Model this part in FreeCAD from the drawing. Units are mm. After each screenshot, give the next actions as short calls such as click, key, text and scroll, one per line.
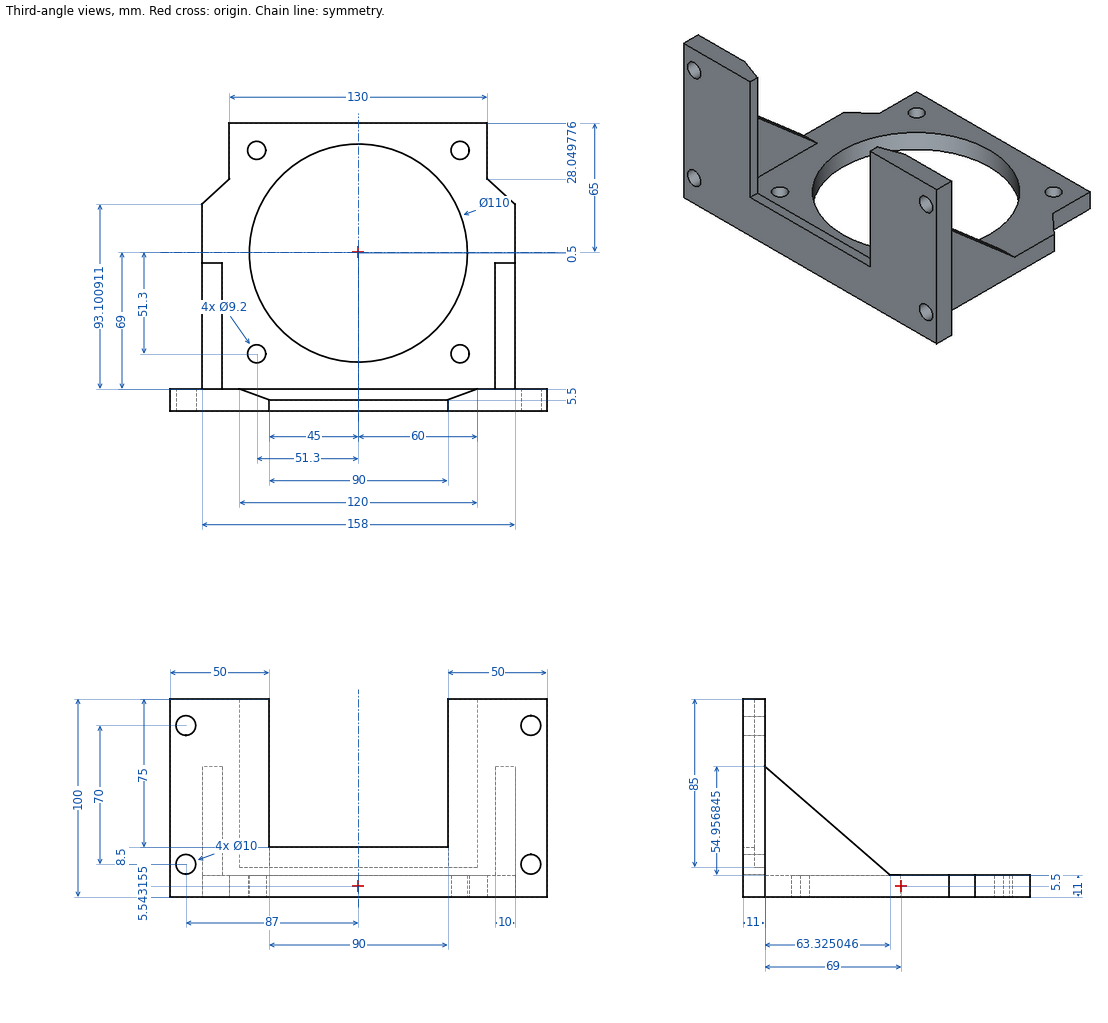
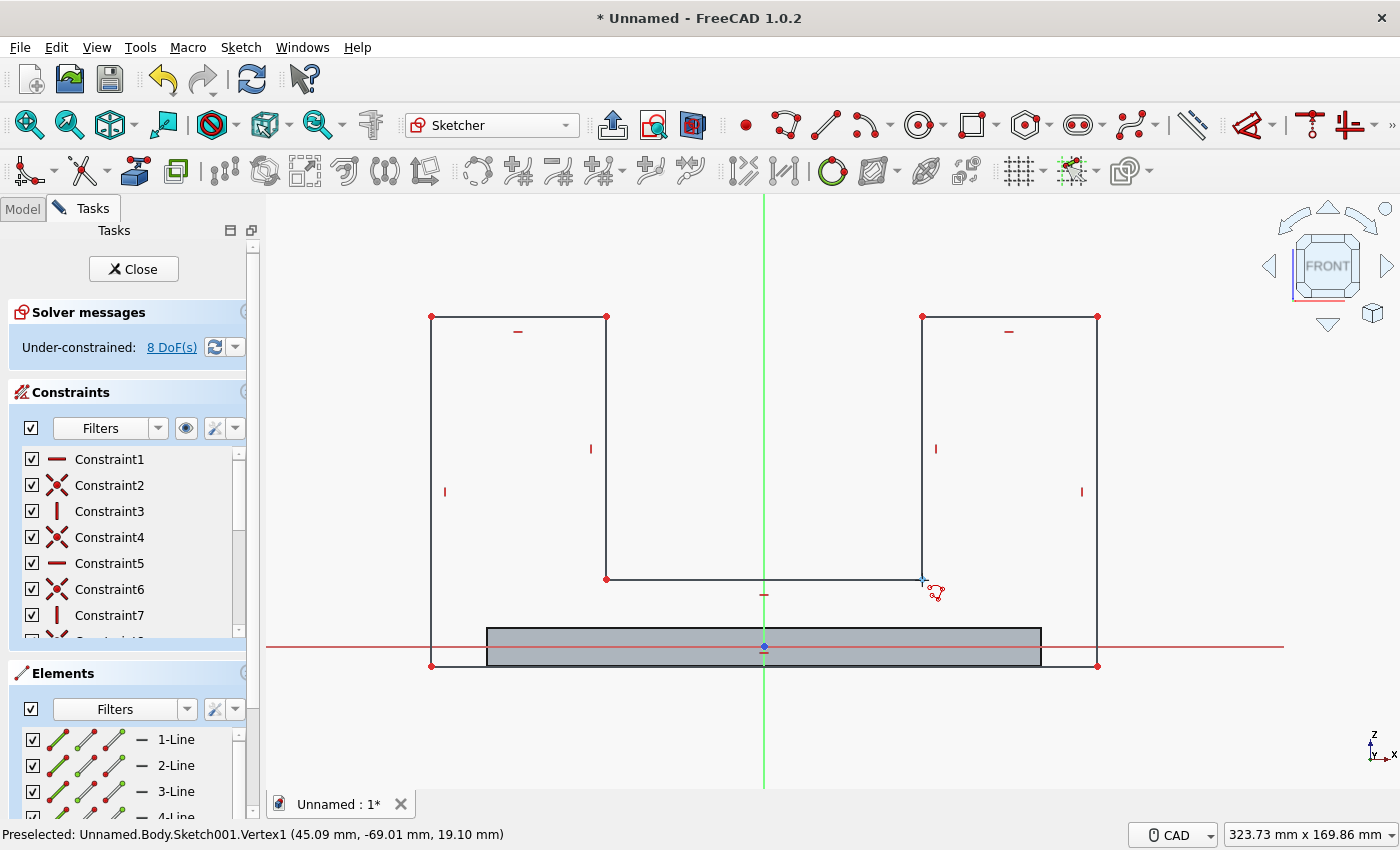
key(g)
key(c)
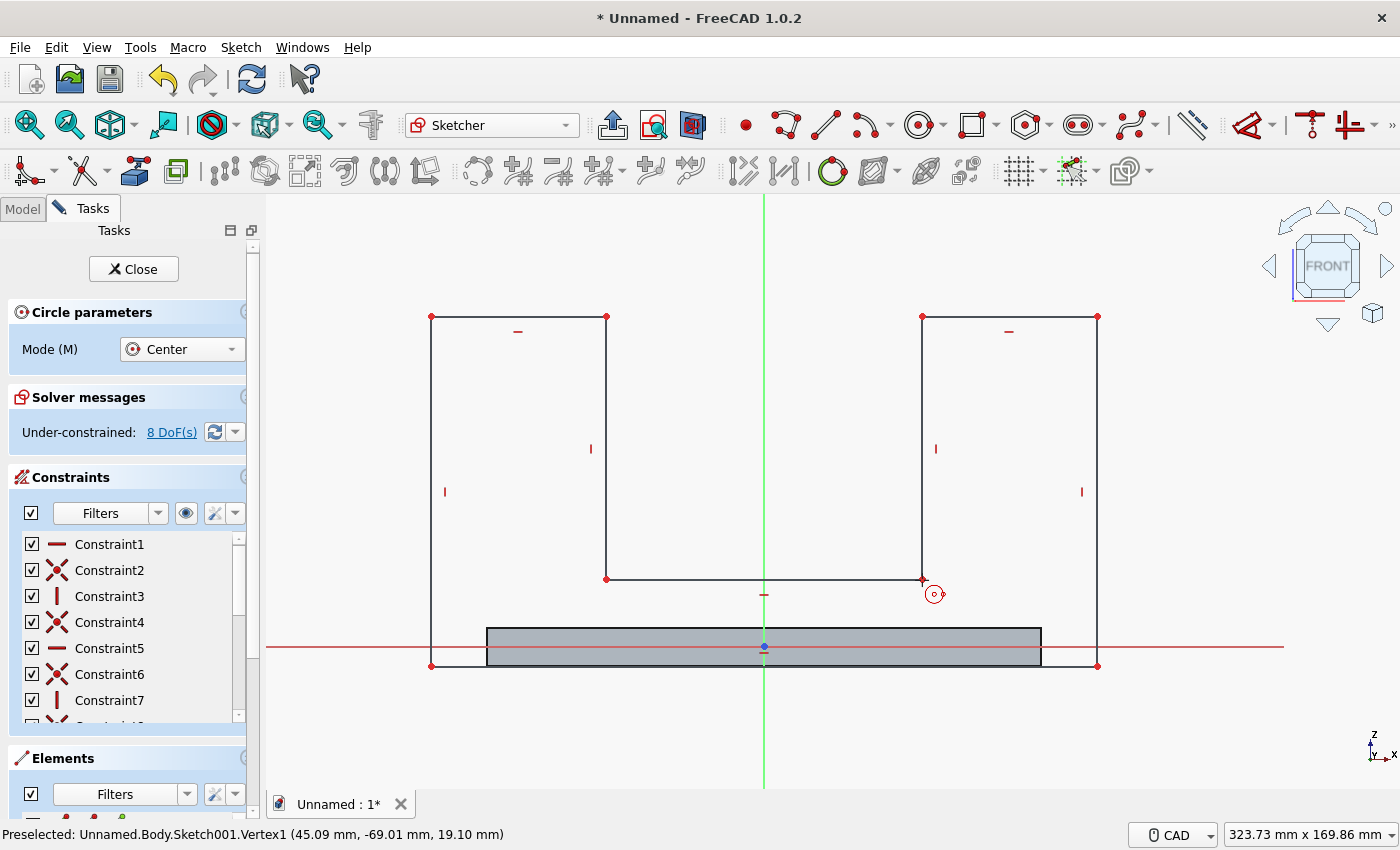
scroll(459, 609, up, 2)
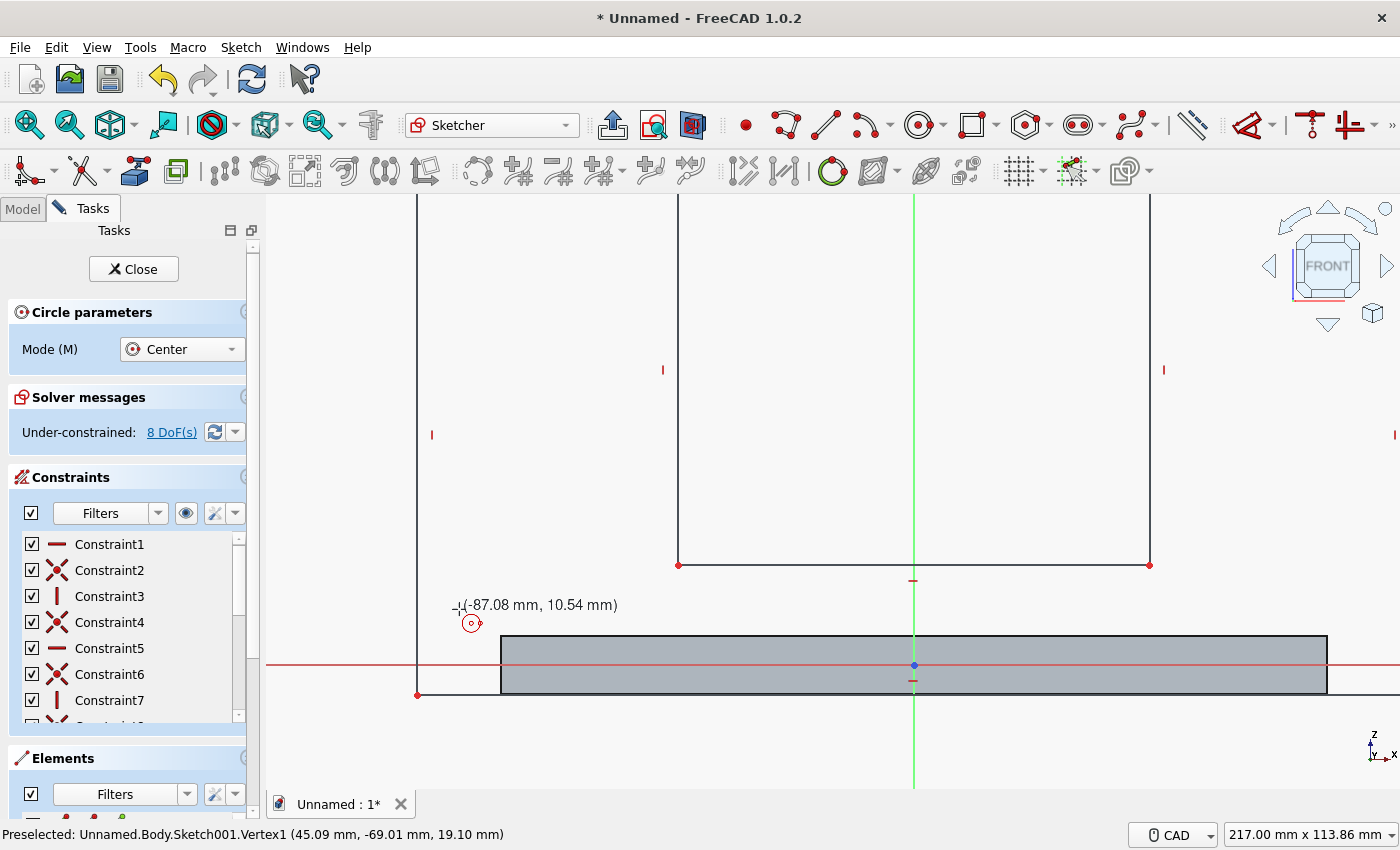
click(459, 608)
move(478, 589)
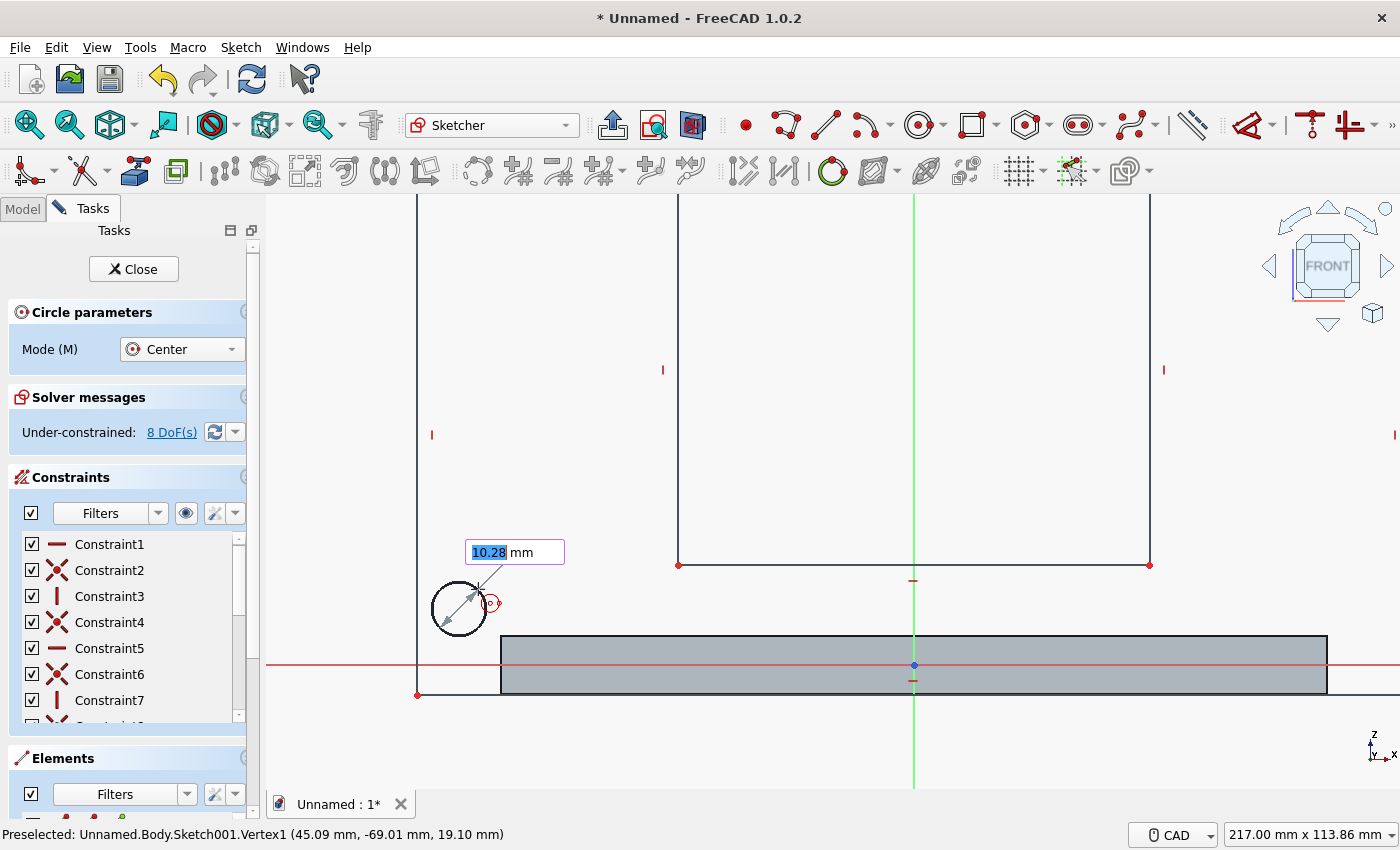
text(10)
key(Return)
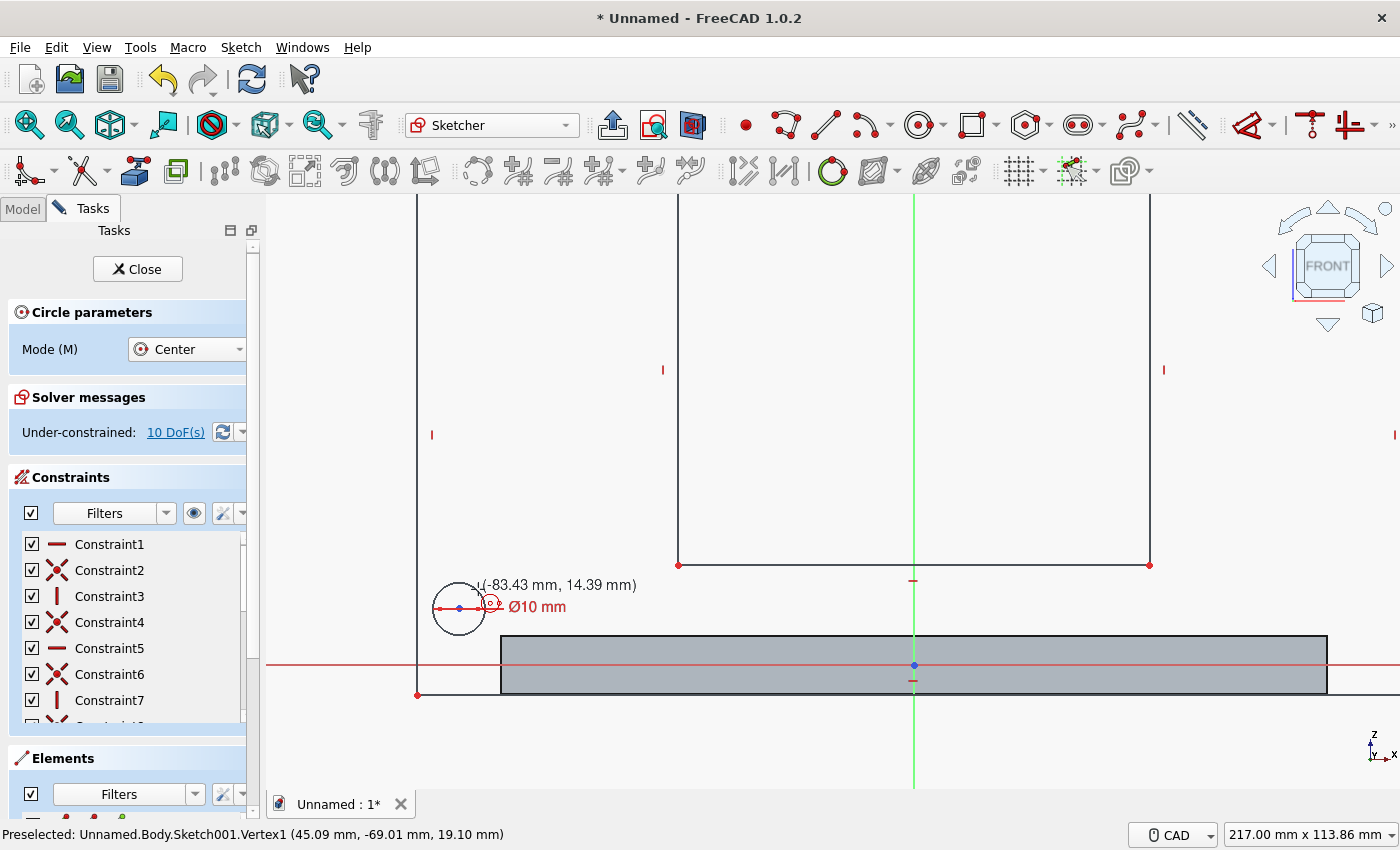
scroll(461, 611, down, 2)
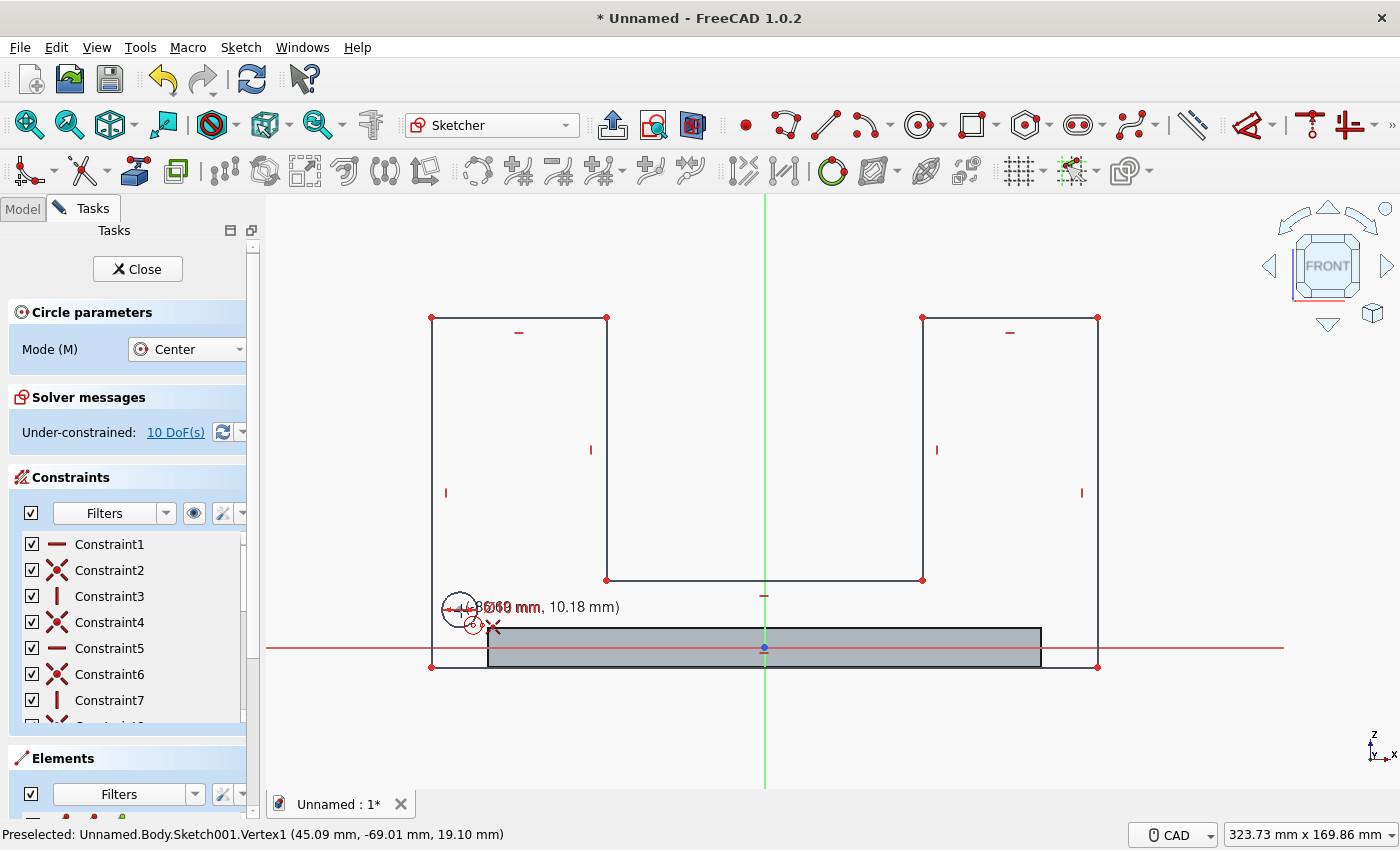
scroll(1069, 609, up, 2)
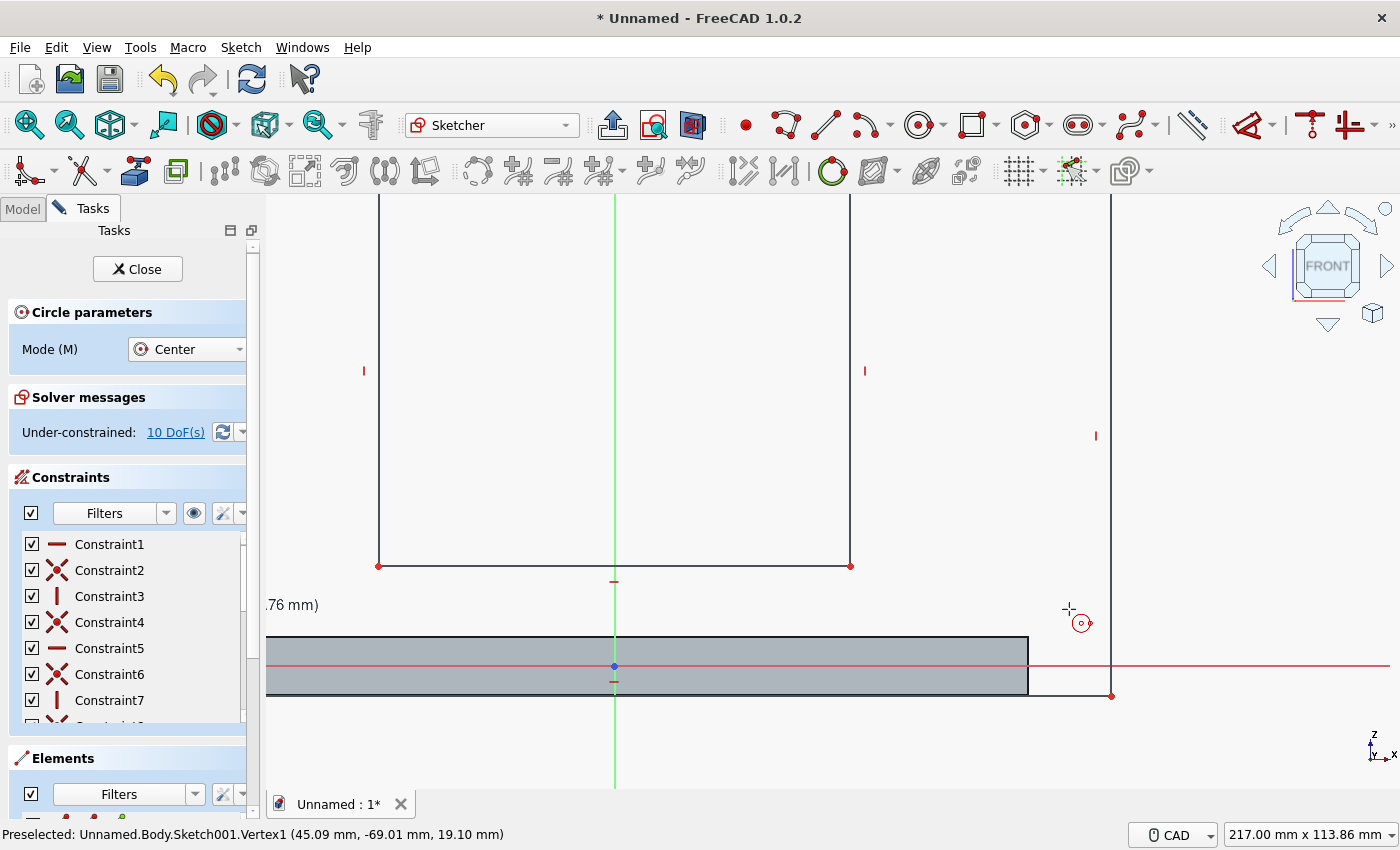
click(1069, 609)
move(1088, 590)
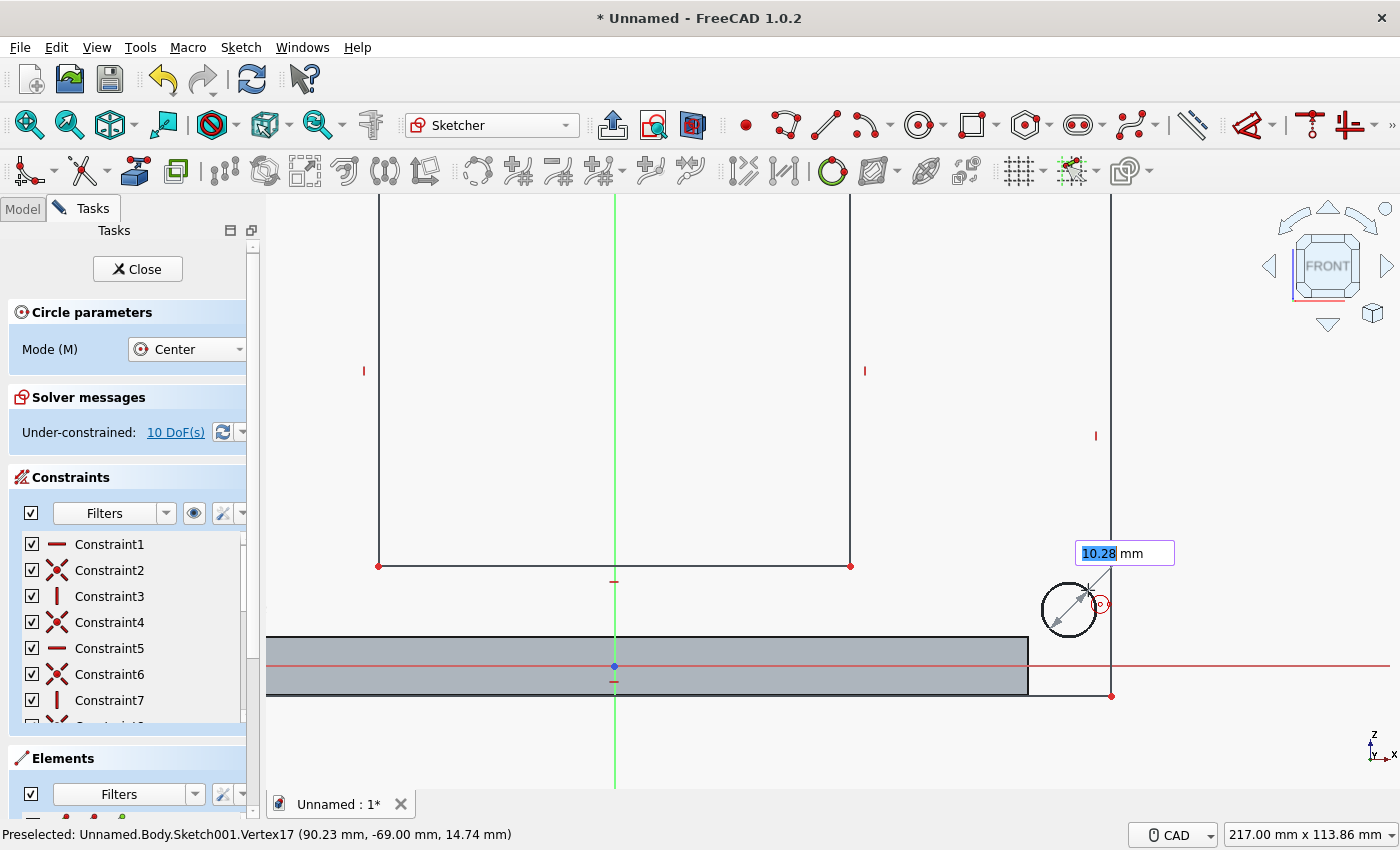
text(10)
key(Return)